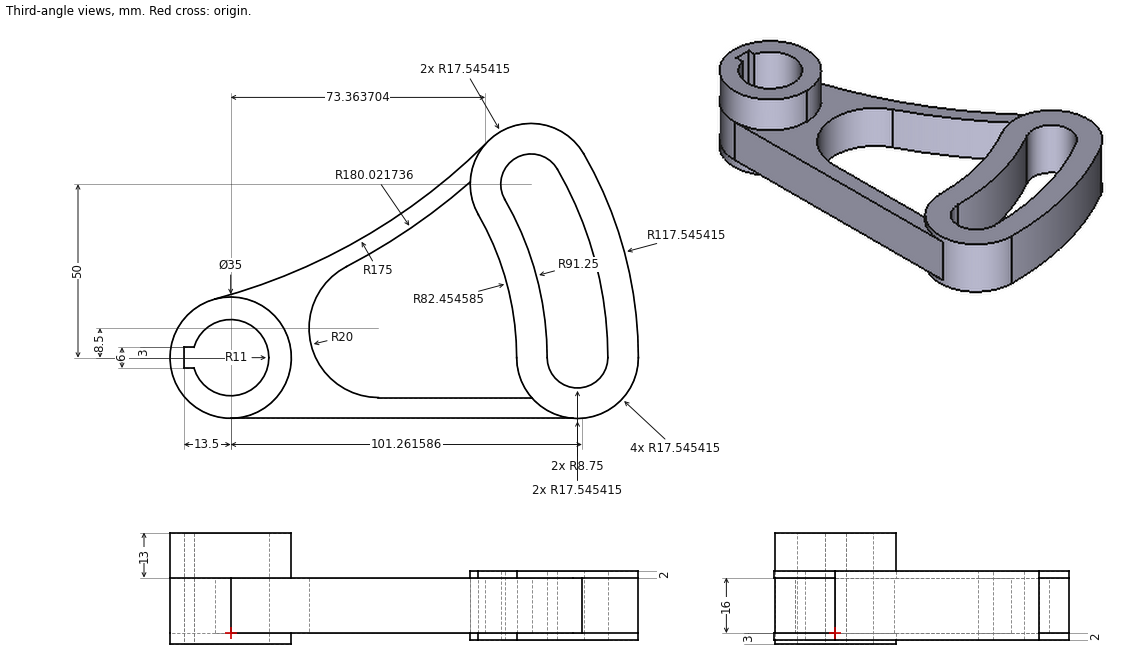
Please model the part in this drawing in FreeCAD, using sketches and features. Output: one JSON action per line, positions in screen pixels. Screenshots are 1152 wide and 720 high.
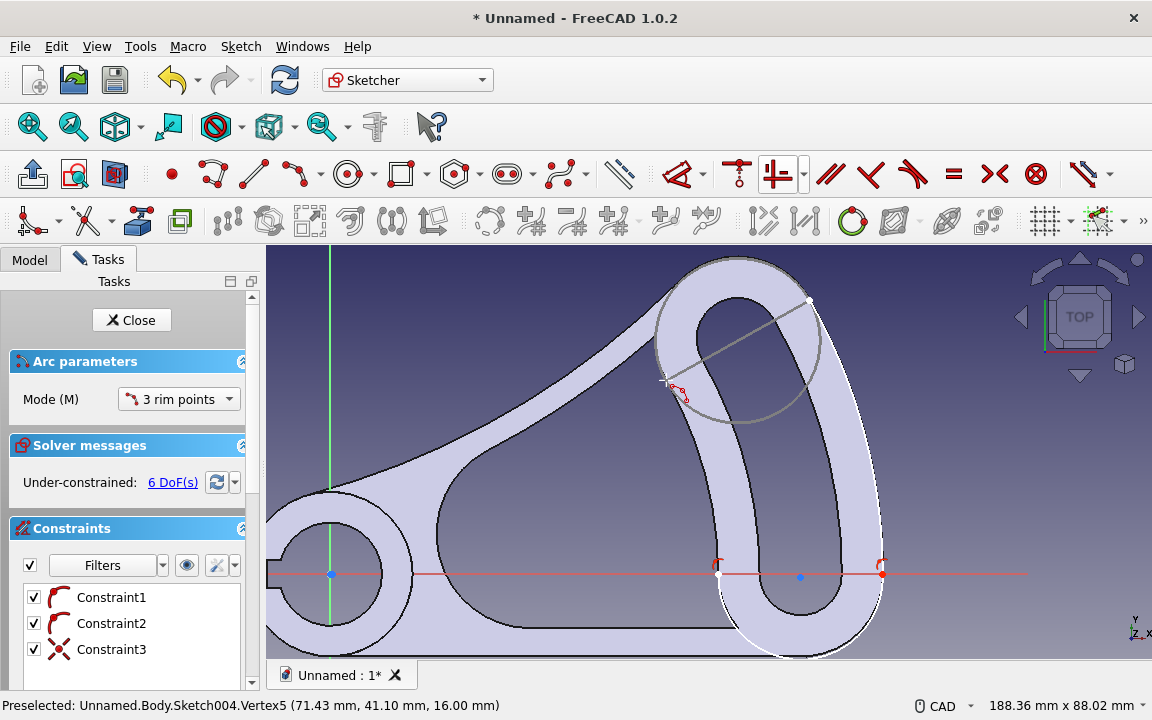
{"action": "scroll", "coordinate": [709, 431], "scroll_direction": "down", "scroll_amount": 2}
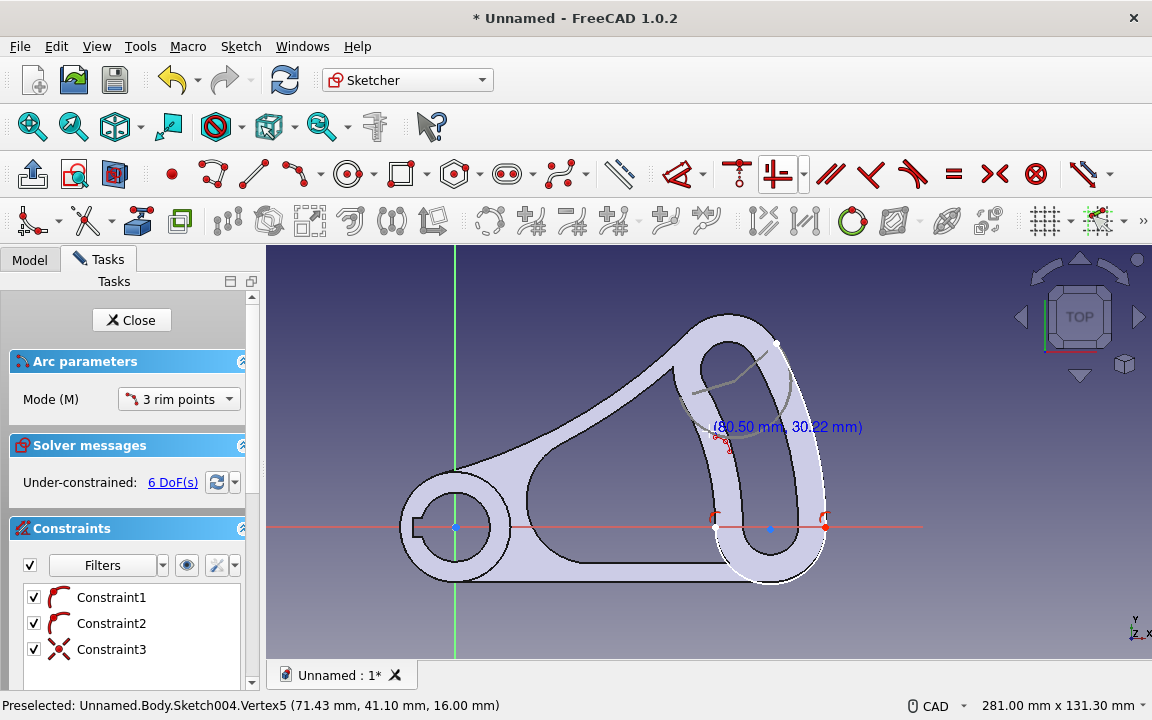
{"action": "left_click", "coordinate": [701, 322]}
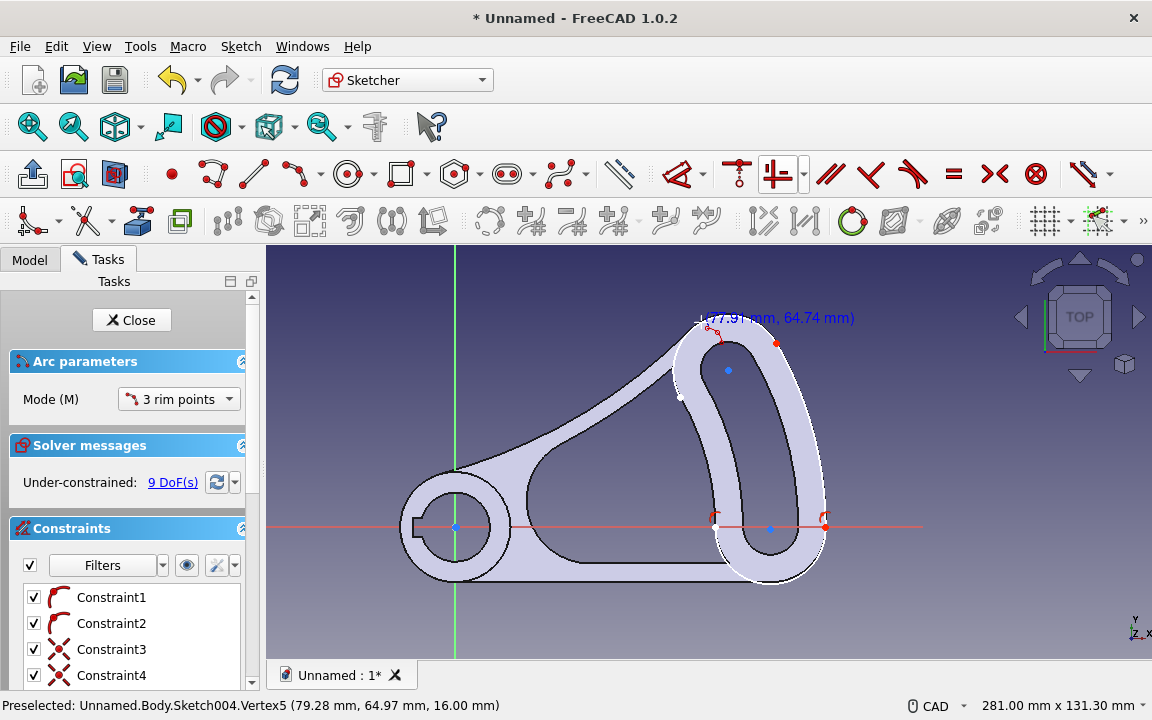
{"action": "left_click", "coordinate": [680, 398]}
{"action": "left_click", "coordinate": [716, 527]}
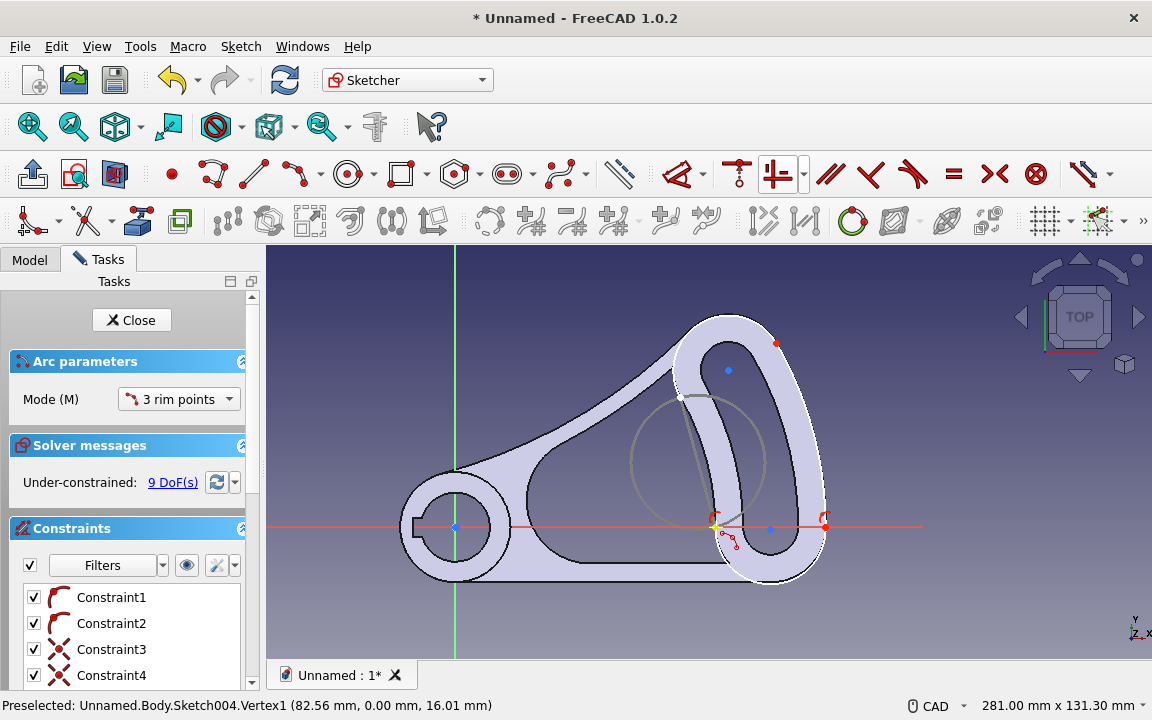
{"action": "scroll", "coordinate": [706, 460], "scroll_direction": "up", "scroll_amount": 3}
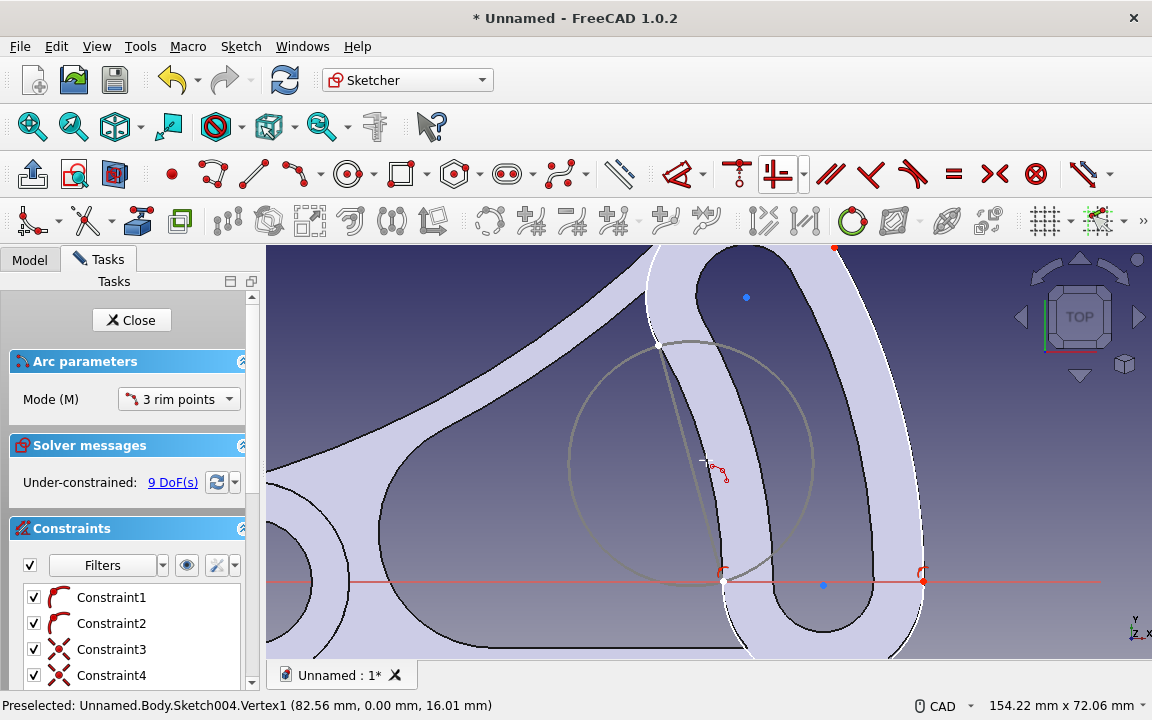
{"action": "left_click", "coordinate": [706, 459]}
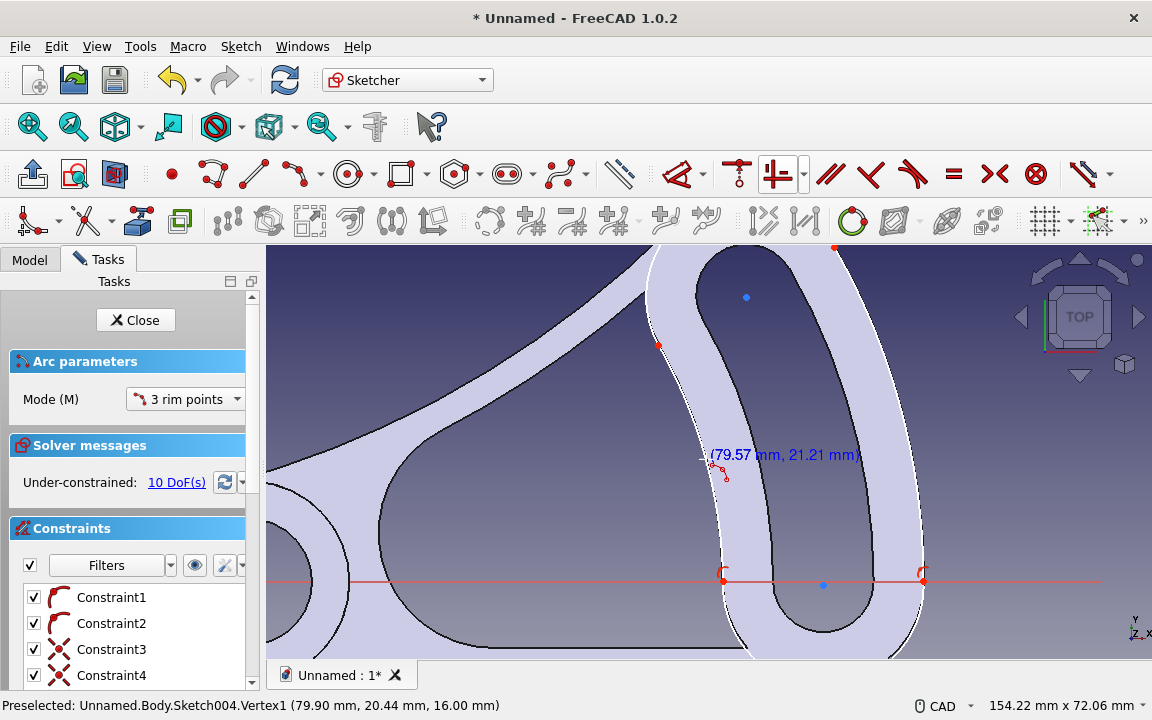
{"action": "left_click", "coordinate": [703, 320]}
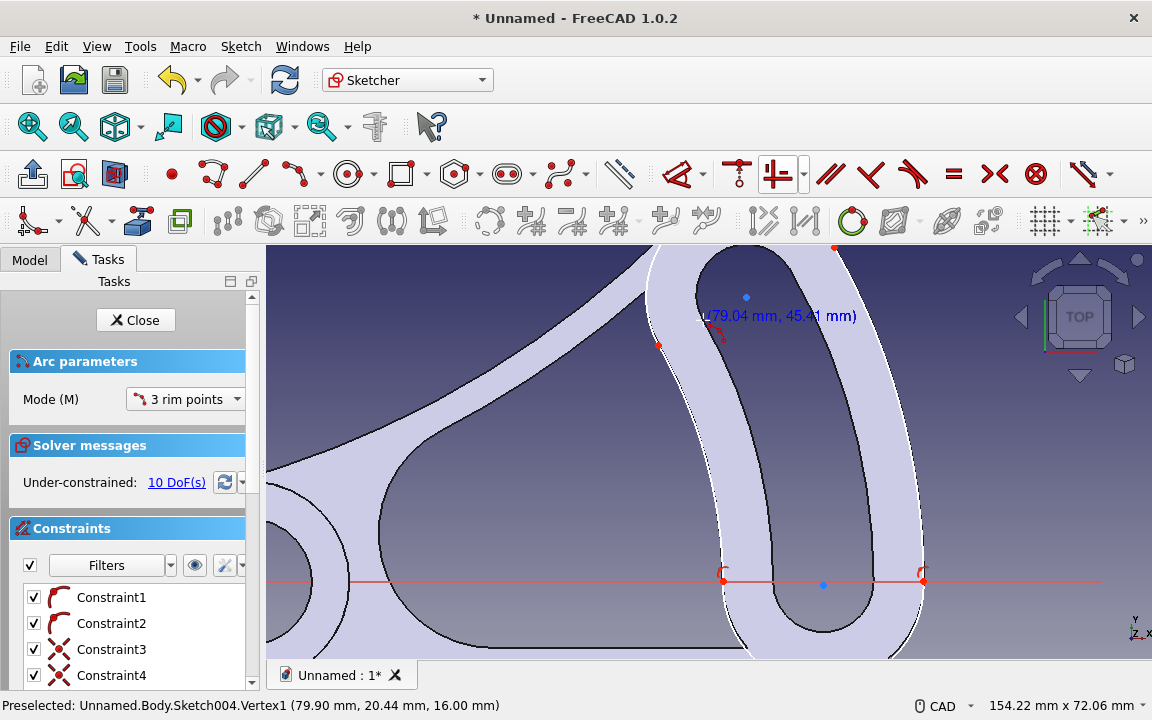
{"action": "scroll", "coordinate": [706, 461], "scroll_direction": "down", "scroll_amount": 3}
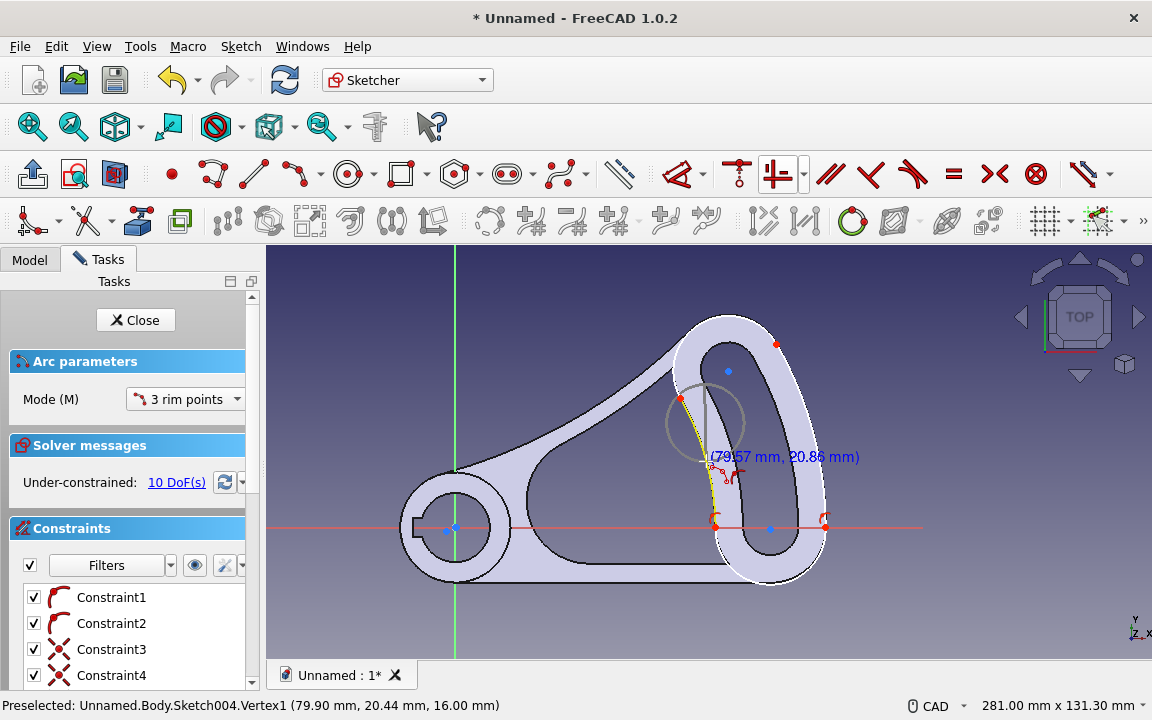
{"action": "left_click", "coordinate": [752, 356]}
{"action": "left_click", "coordinate": [715, 346]}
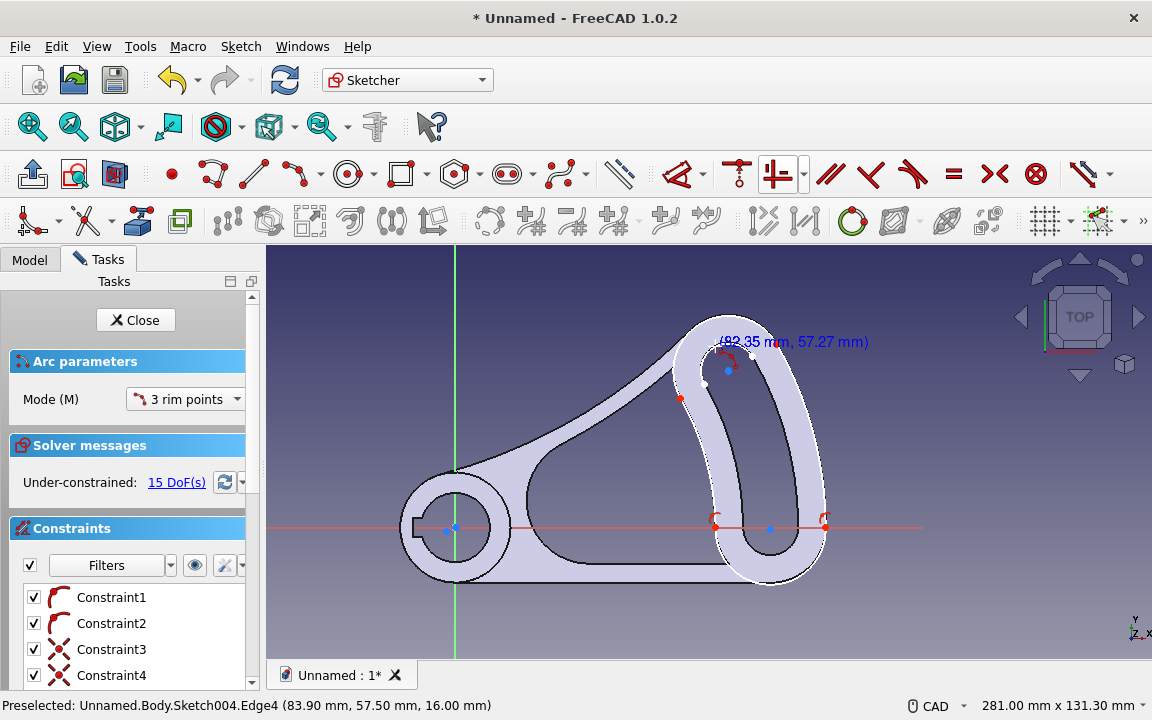
{"action": "left_click", "coordinate": [752, 357]}
{"action": "left_click", "coordinate": [798, 528]}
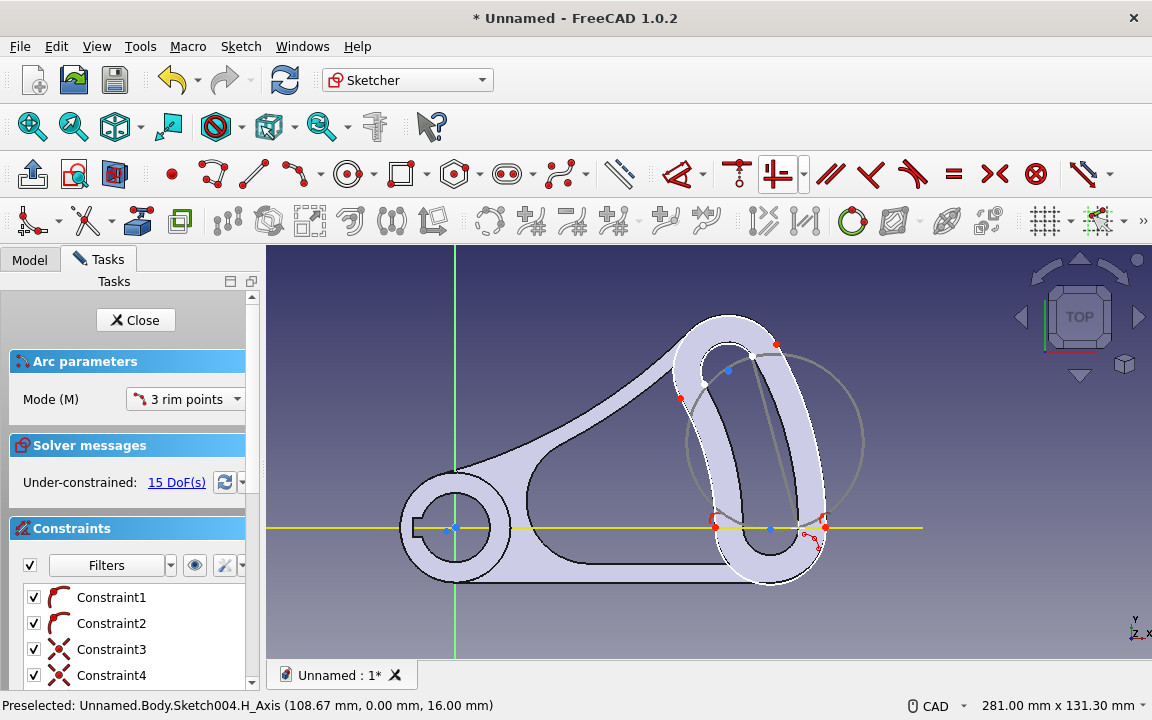
{"action": "scroll", "coordinate": [787, 439], "scroll_direction": "up", "scroll_amount": 2}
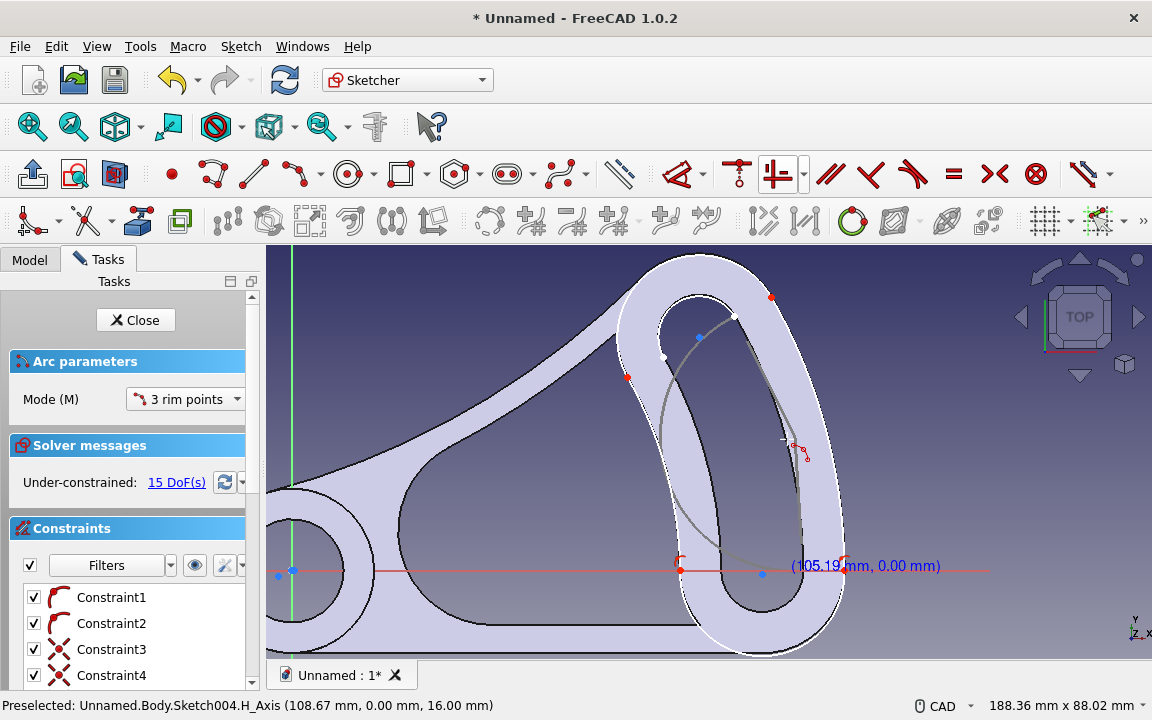
{"action": "left_click", "coordinate": [786, 439]}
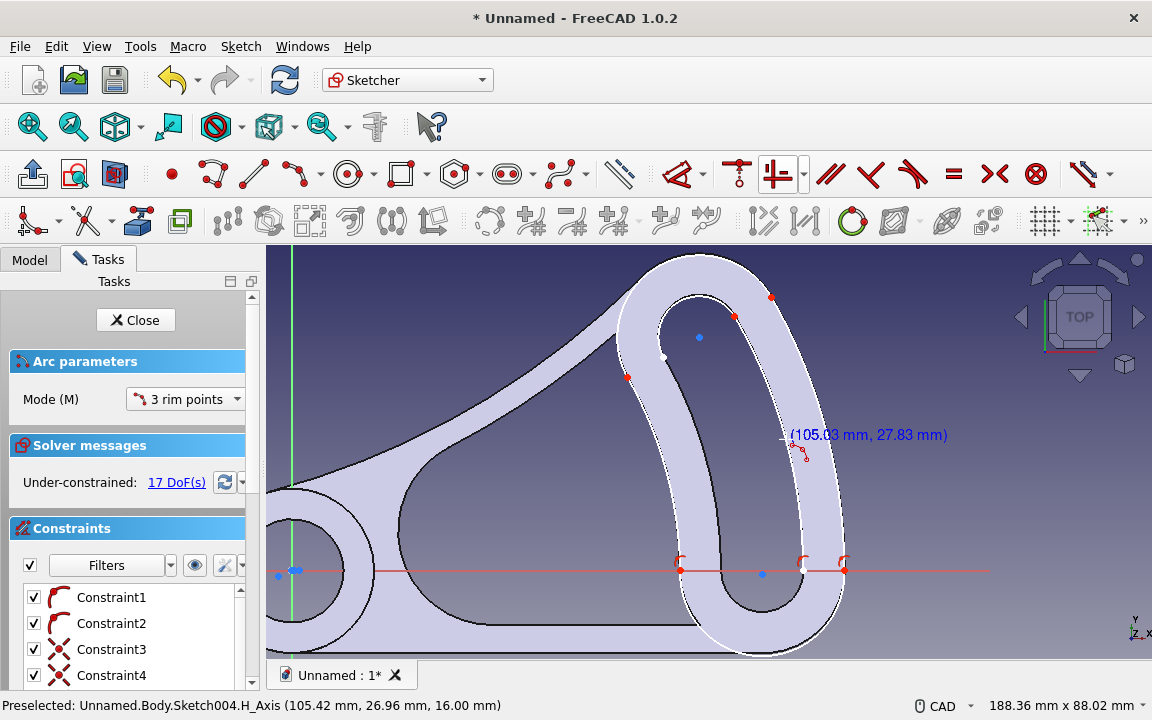
{"action": "left_click", "coordinate": [803, 571]}
{"action": "left_click", "coordinate": [721, 571]}
{"action": "left_click", "coordinate": [762, 612]}